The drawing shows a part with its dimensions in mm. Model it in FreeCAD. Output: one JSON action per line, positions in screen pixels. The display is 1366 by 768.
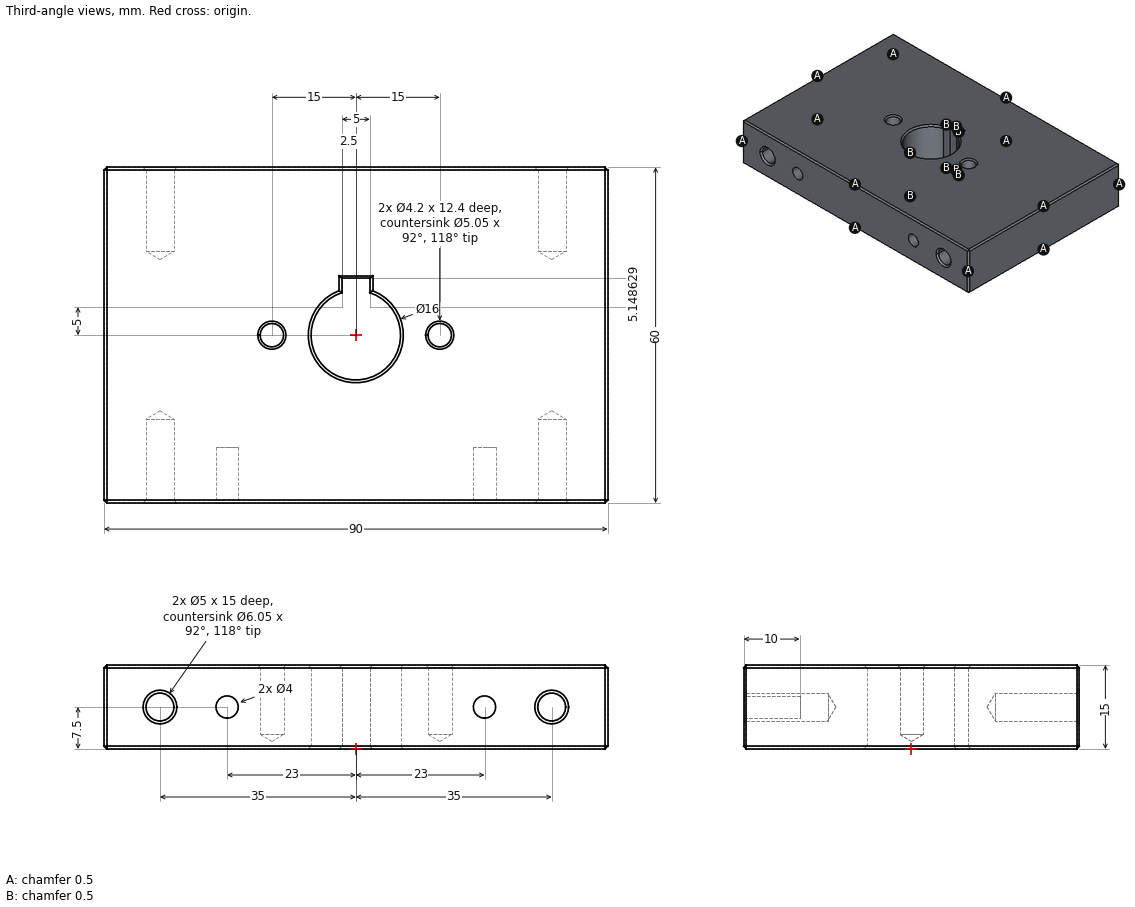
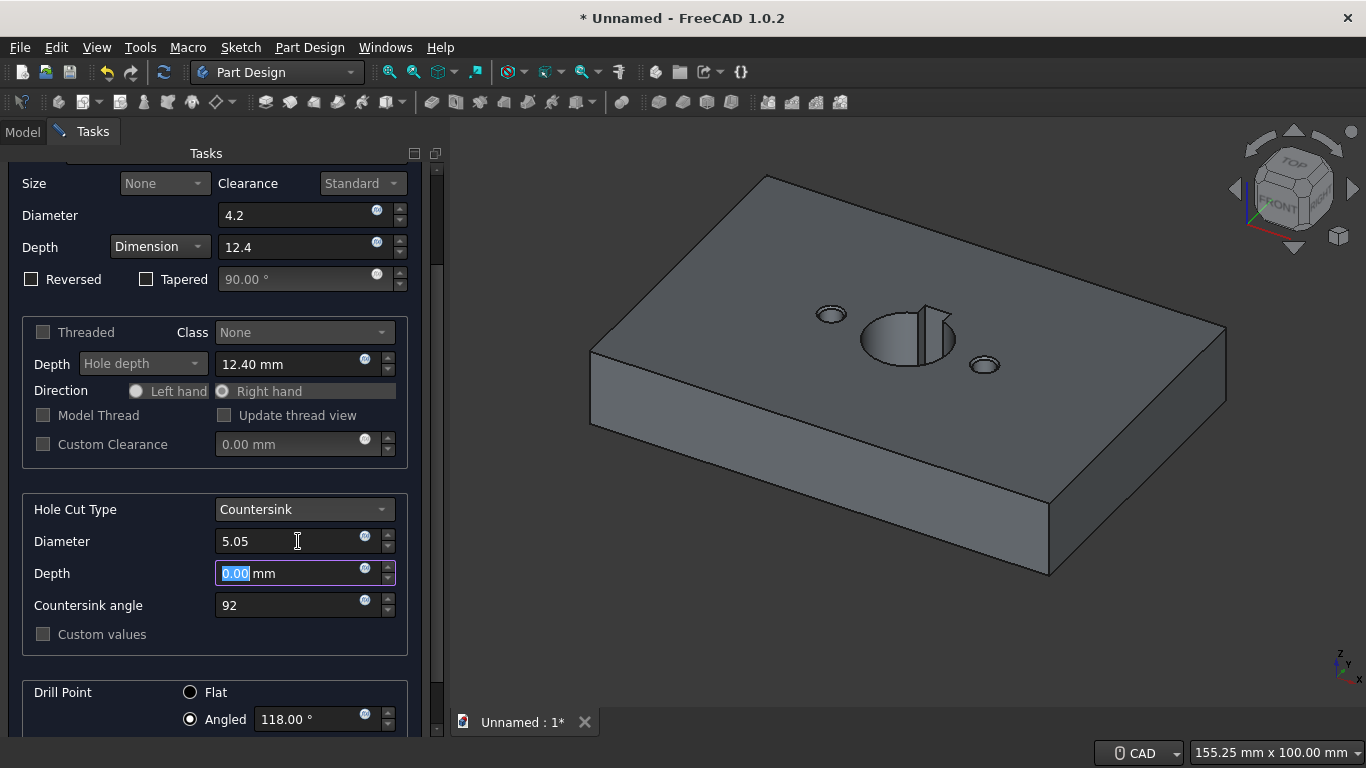
{"action": "scroll", "coordinate": [437, 450], "scroll_direction": "up", "scroll_amount": 3}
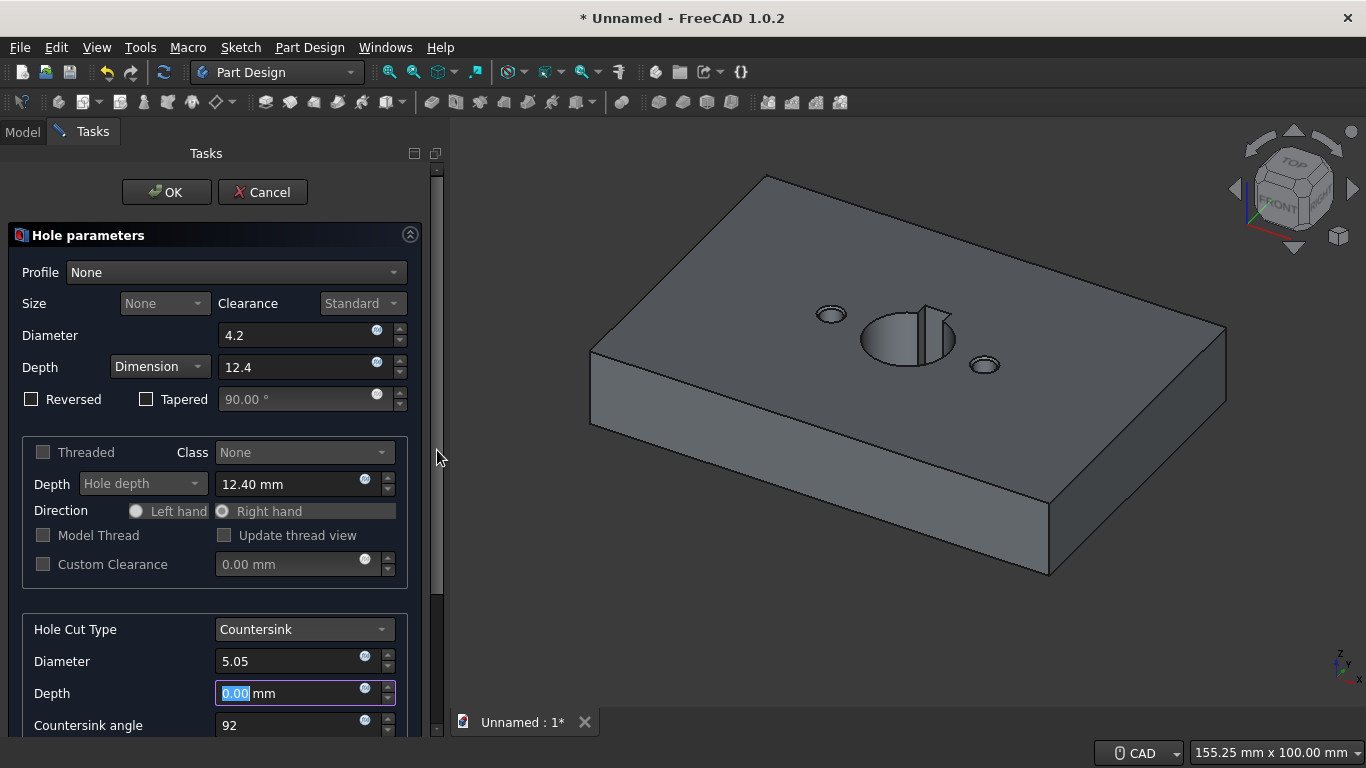
{"action": "left_click", "coordinate": [167, 192]}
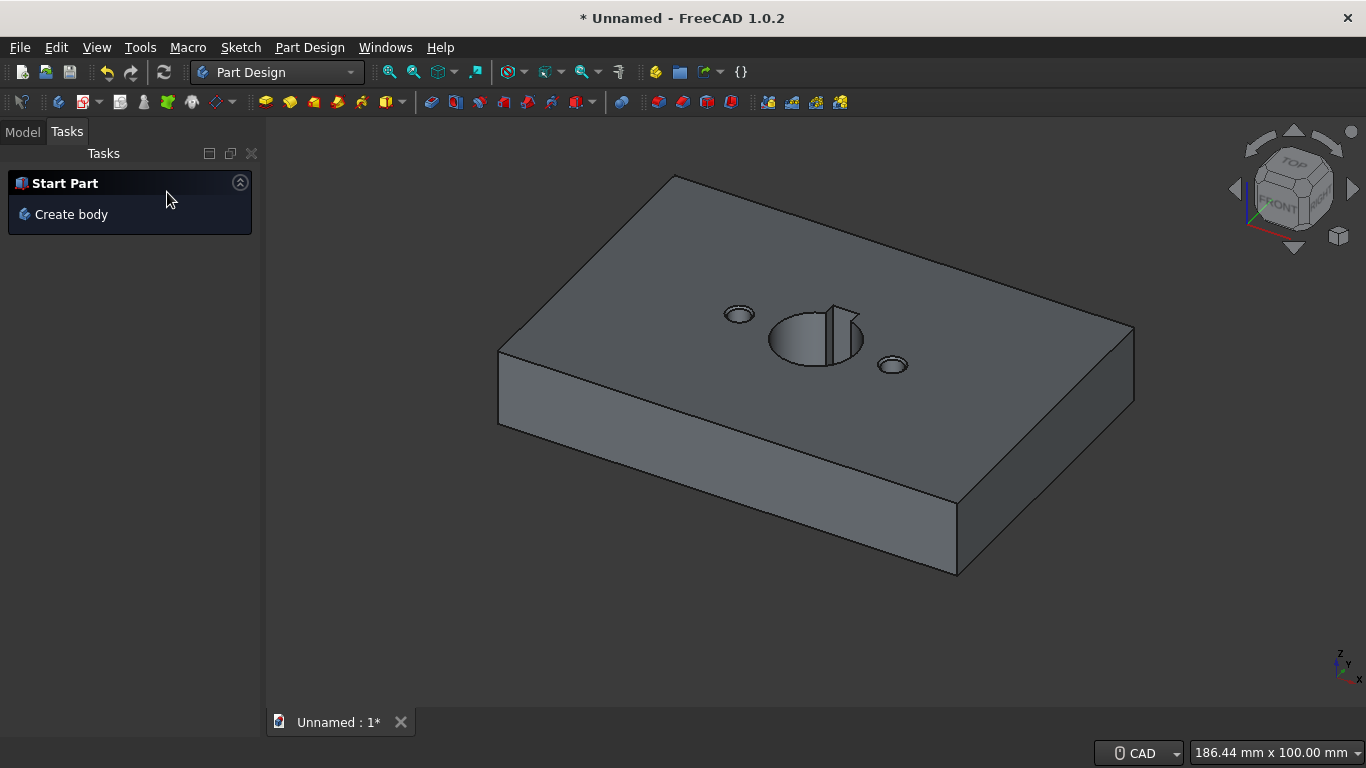
{"action": "left_click", "coordinate": [859, 506]}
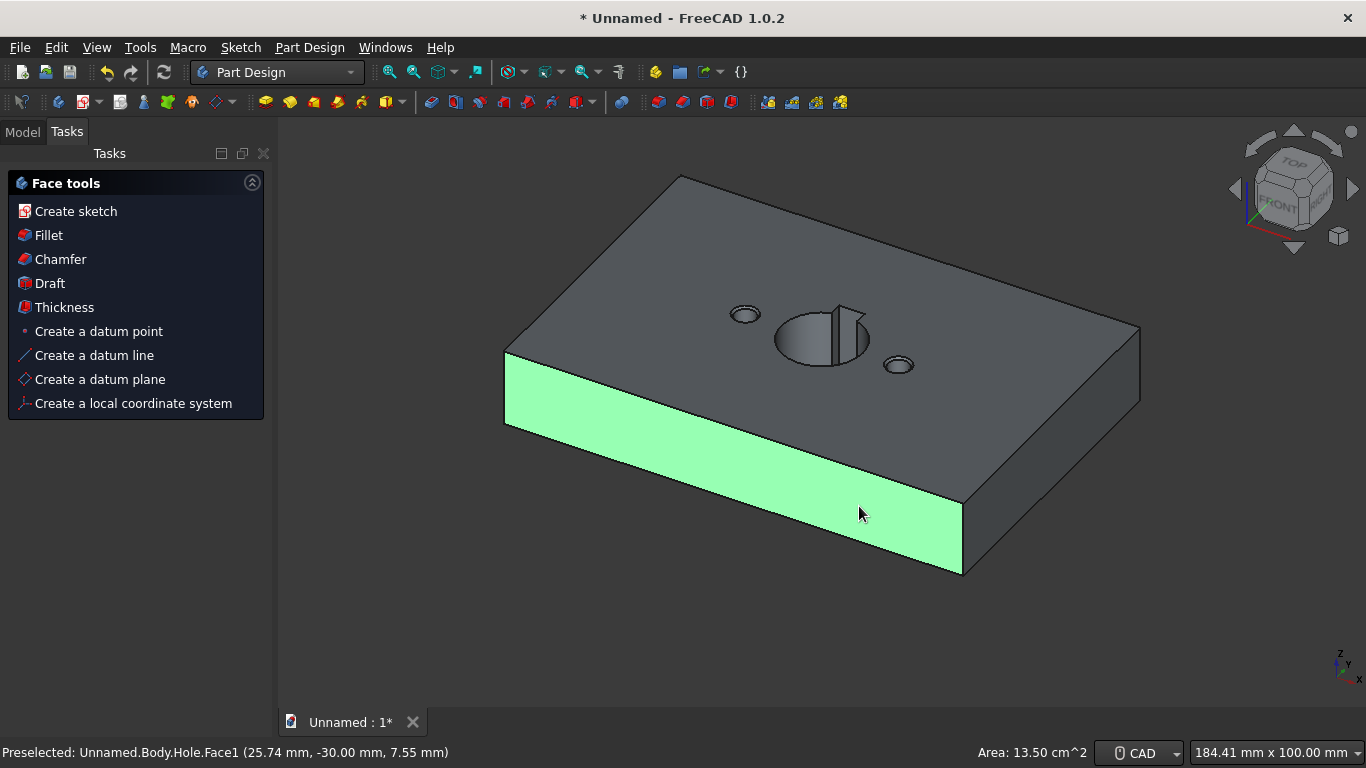
{"action": "left_click", "coordinate": [84, 102]}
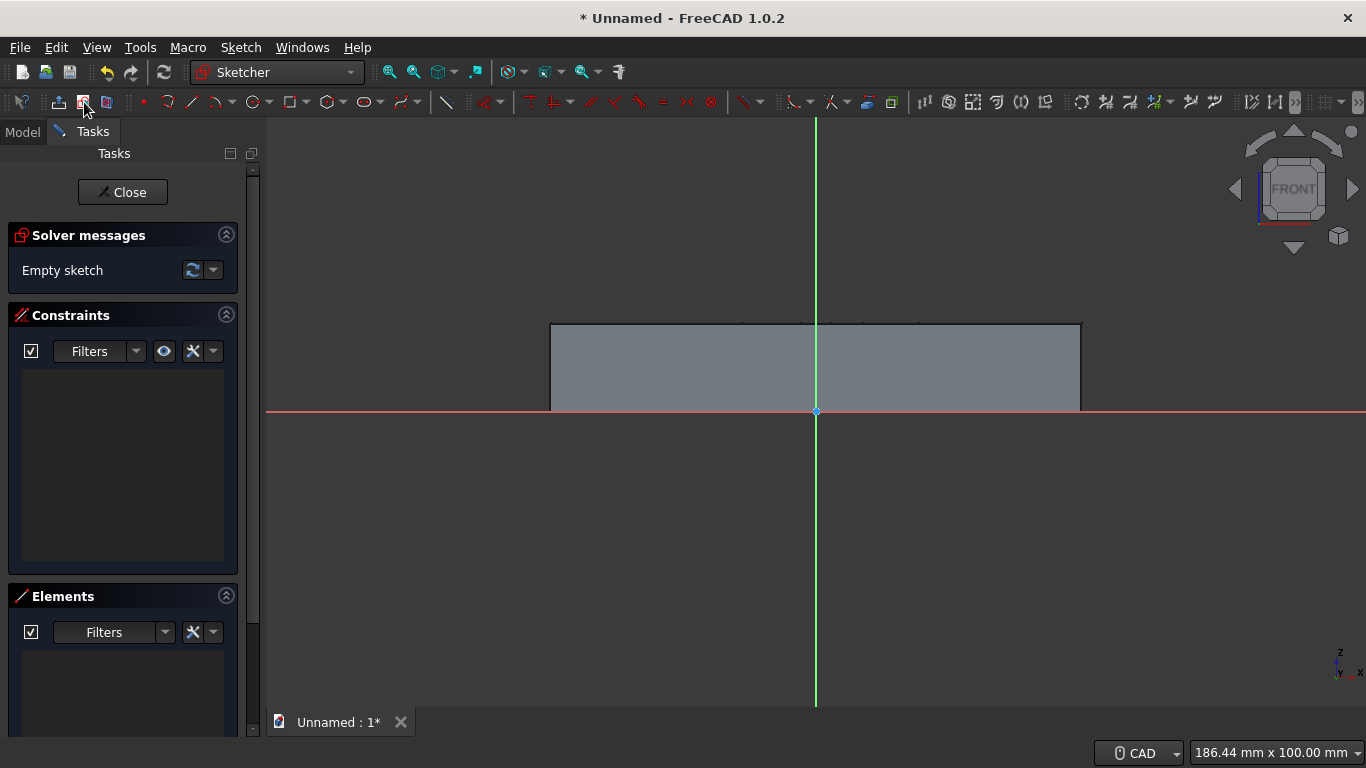
{"action": "scroll", "coordinate": [872, 361], "scroll_direction": "up", "scroll_amount": 4}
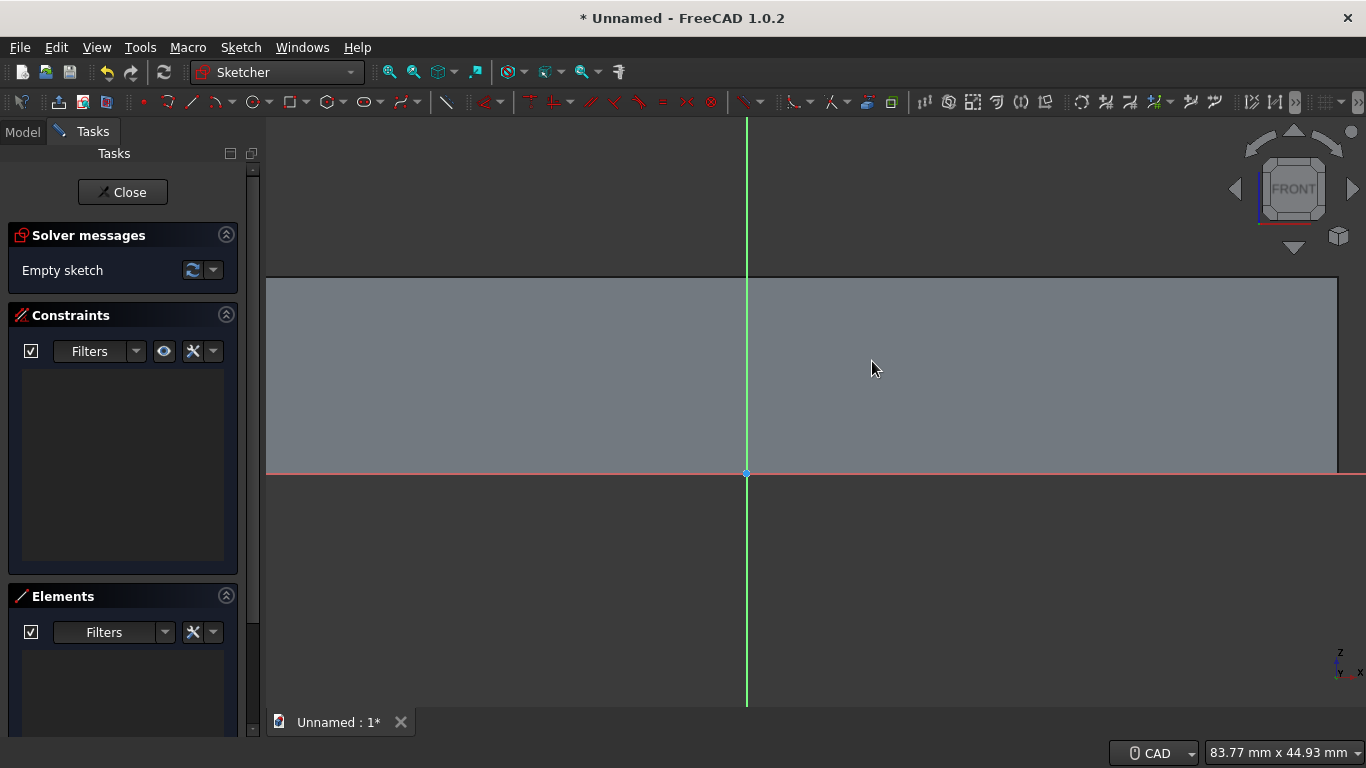
{"action": "key", "text": "g c"}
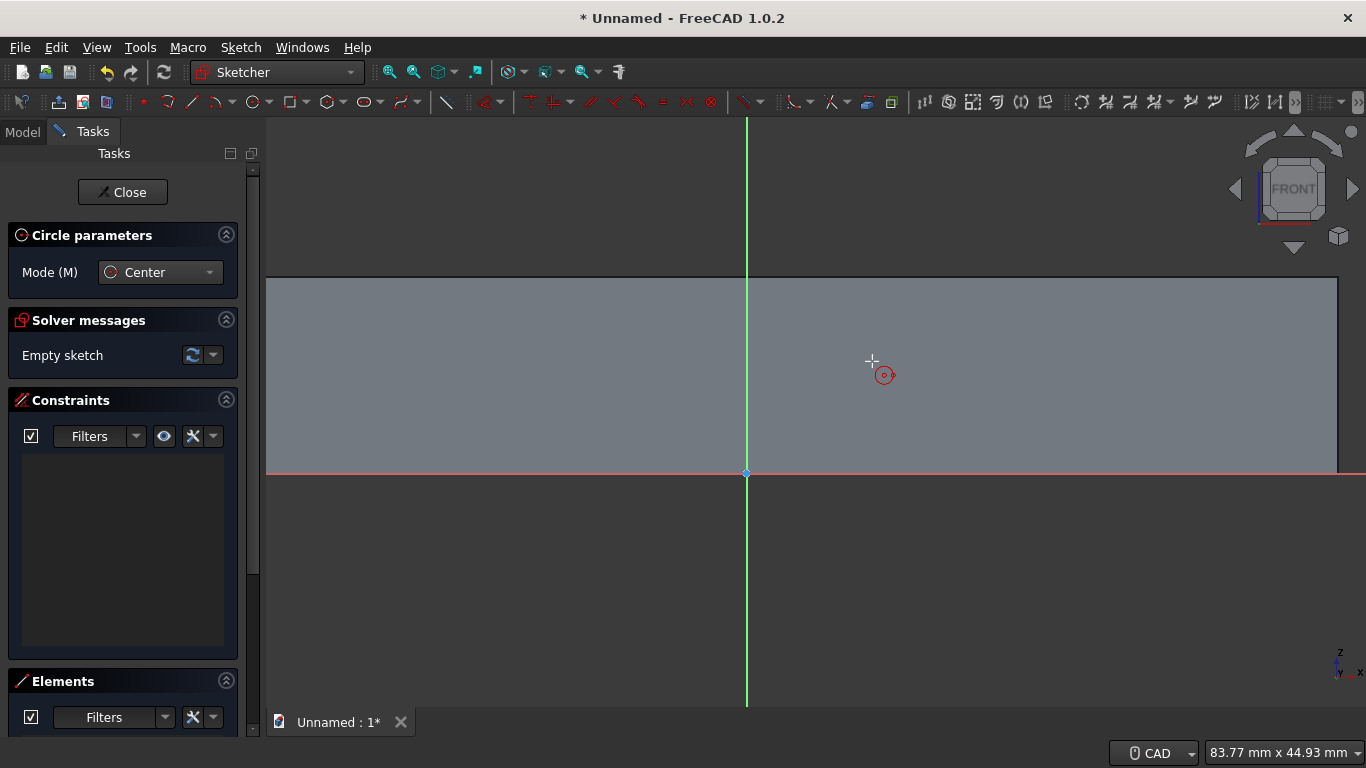
{"action": "left_click", "coordinate": [445, 376]}
{"action": "mouse_move", "coordinate": [463, 357]}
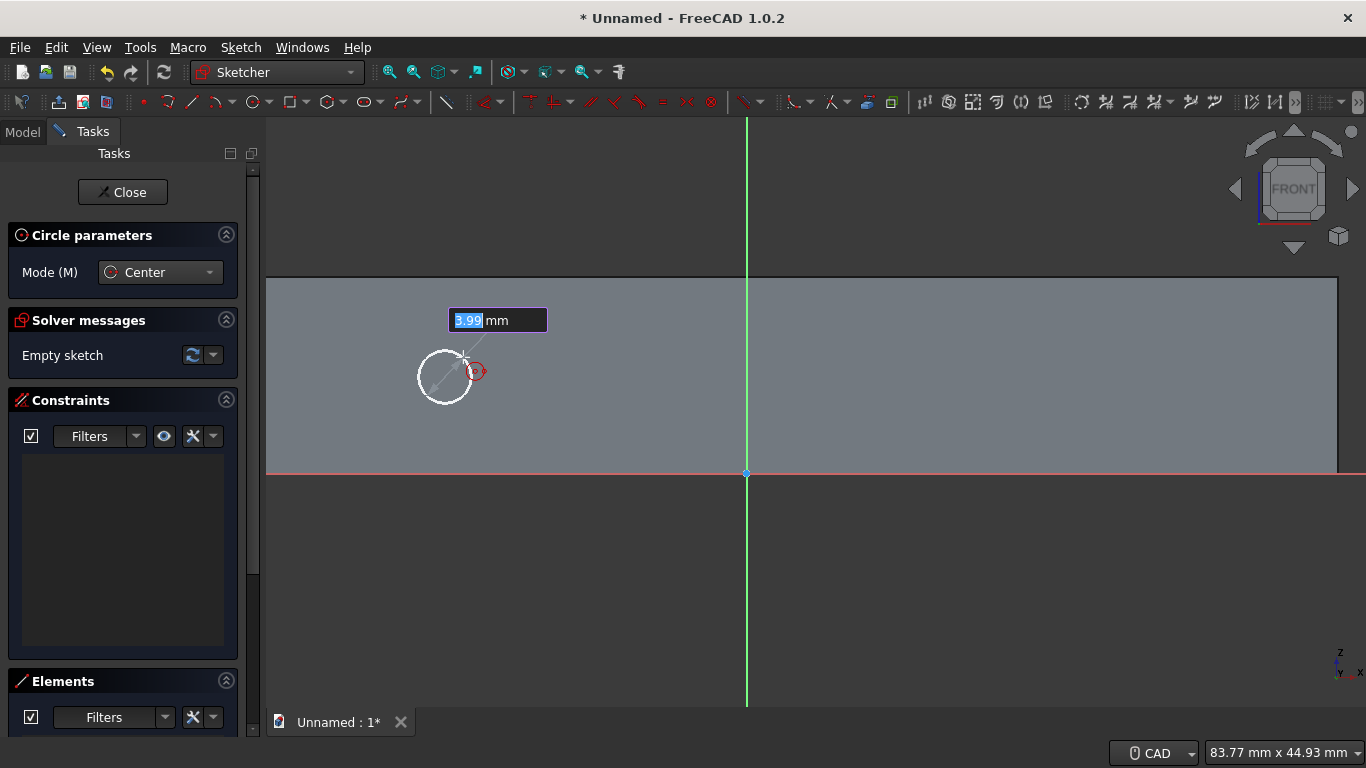
{"action": "type", "text": "4"}
{"action": "key", "text": "Return"}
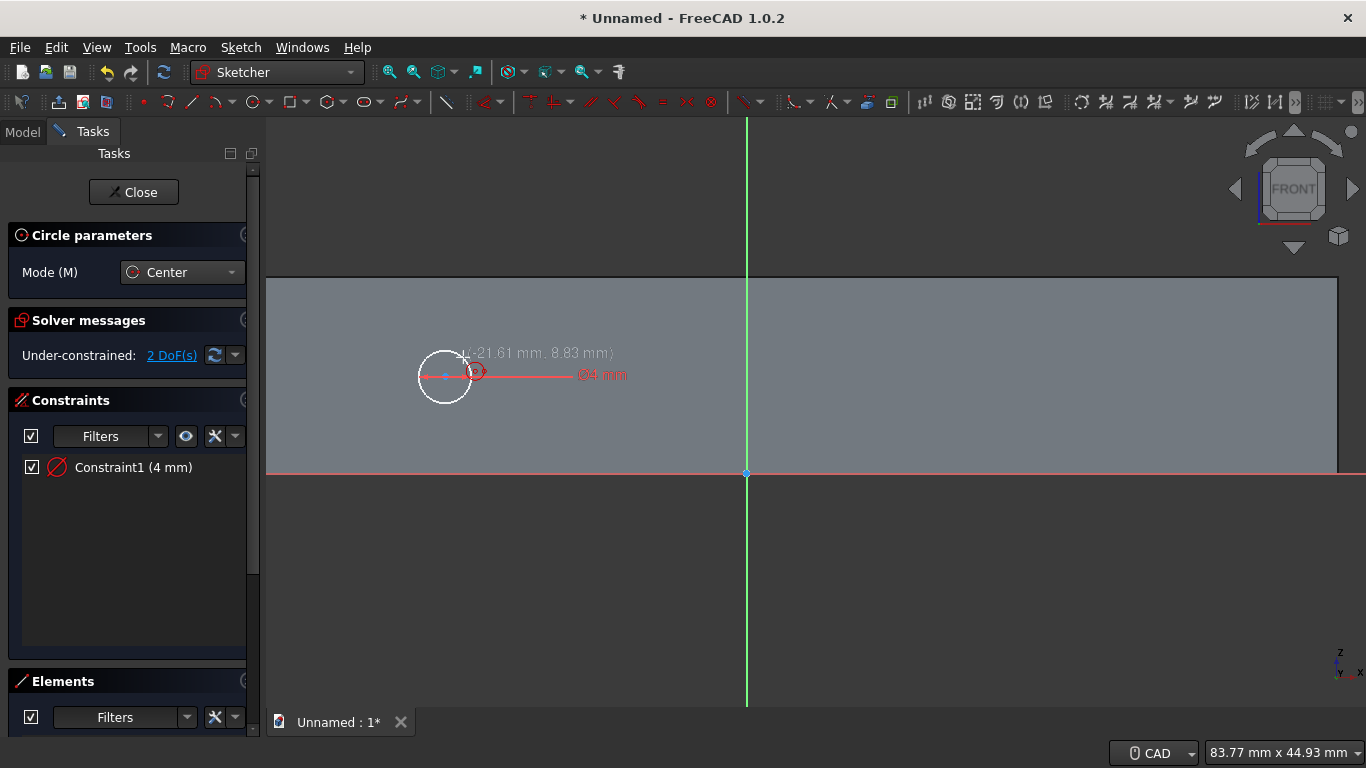
{"action": "left_click", "coordinate": [1049, 376]}
{"action": "mouse_move", "coordinate": [1067, 357]}